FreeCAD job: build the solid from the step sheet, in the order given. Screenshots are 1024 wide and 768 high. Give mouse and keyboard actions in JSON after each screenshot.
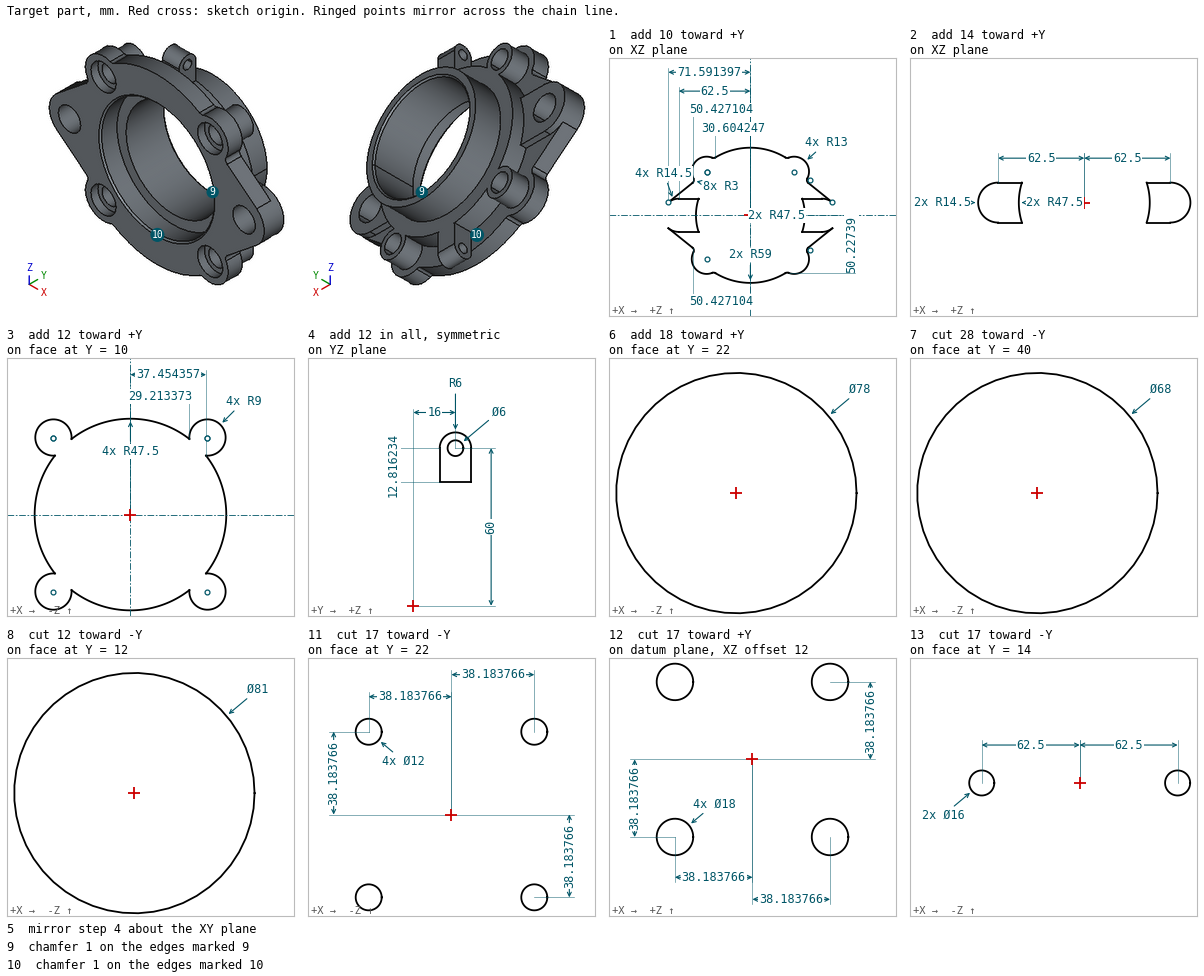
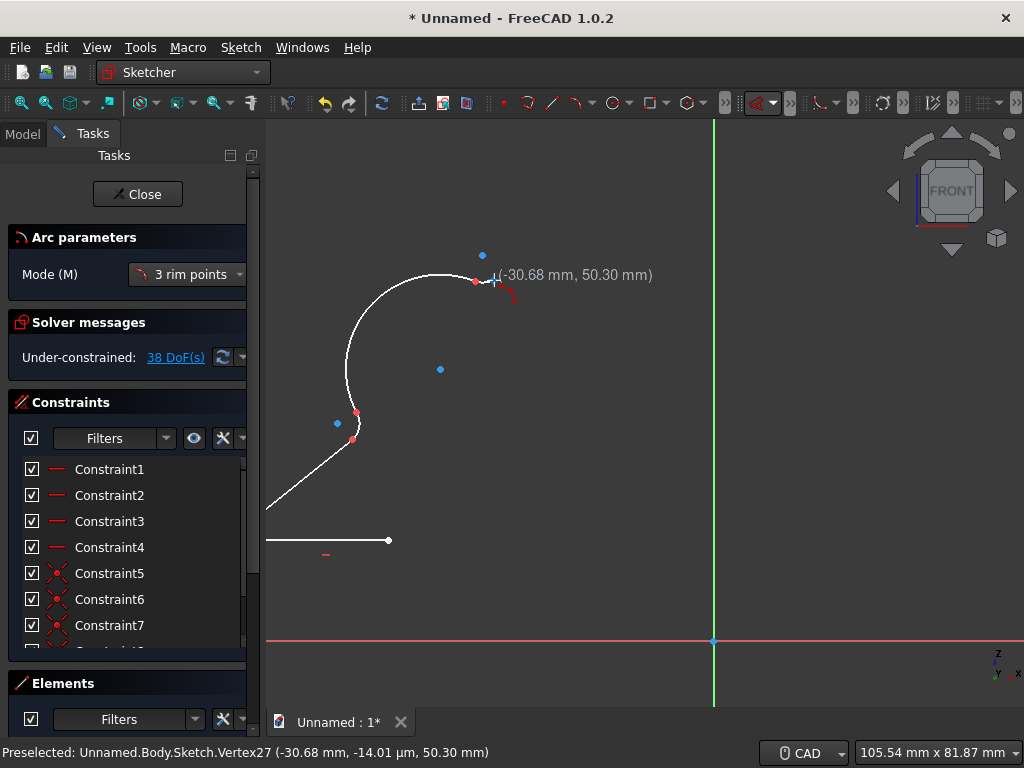
{"action": "scroll", "coordinate": [497, 280], "scroll_direction": "down", "scroll_amount": 5}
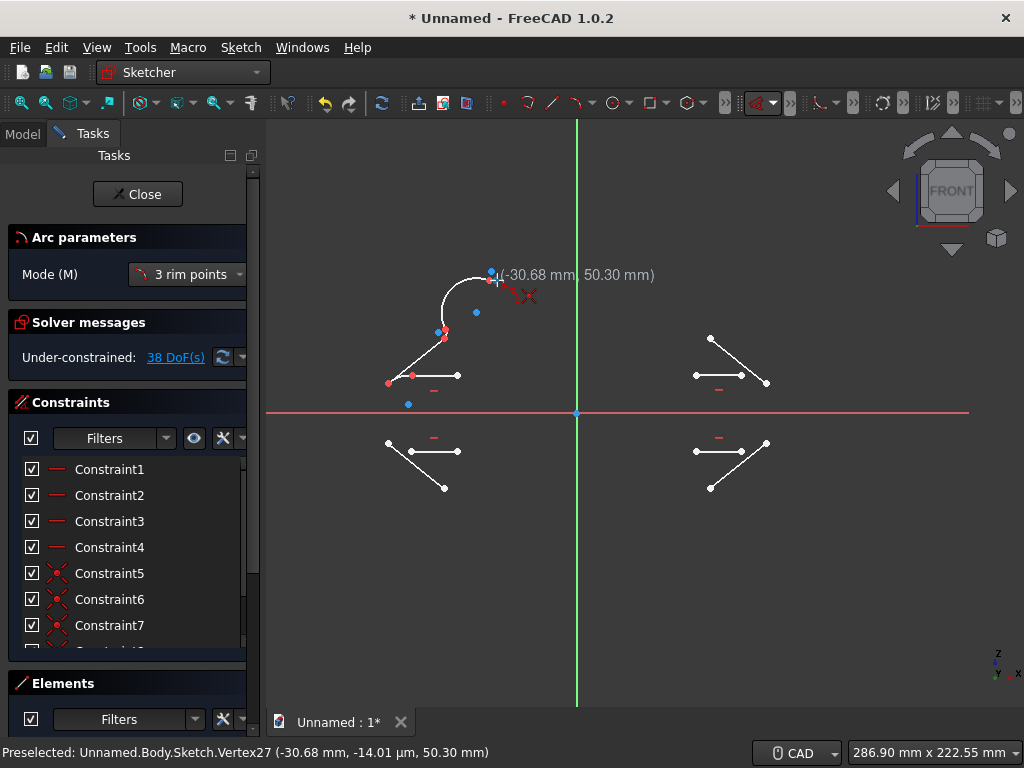
{"action": "left_click", "coordinate": [658, 280]}
{"action": "left_click", "coordinate": [594, 258]}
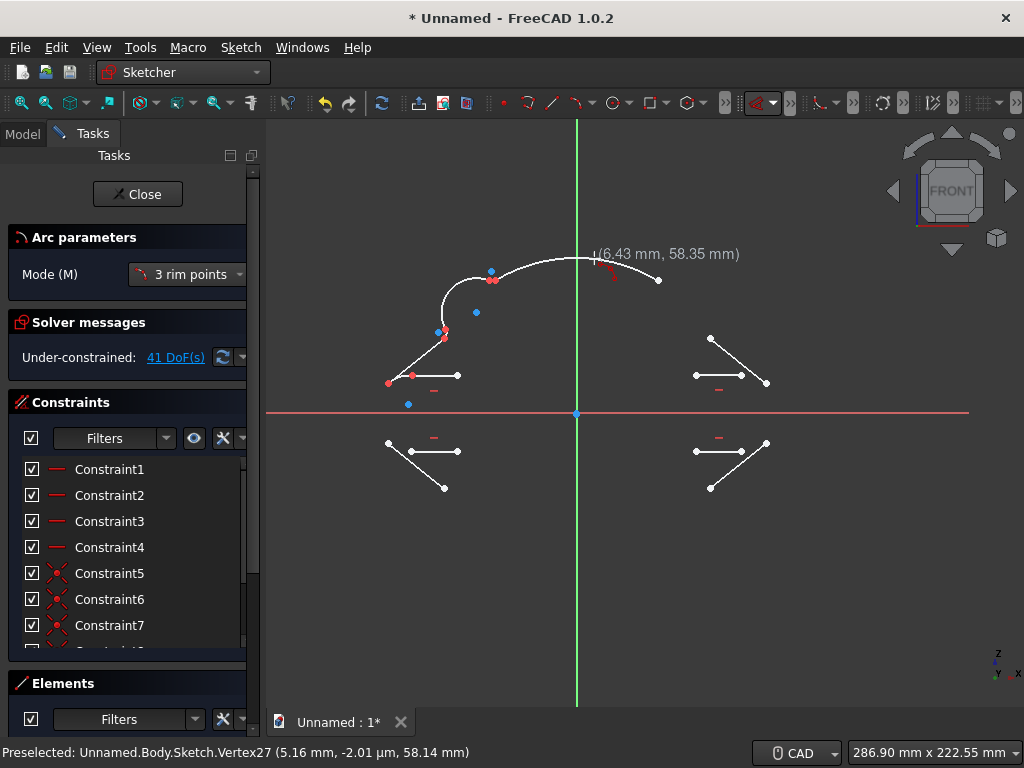
{"action": "left_click", "coordinate": [658, 281]}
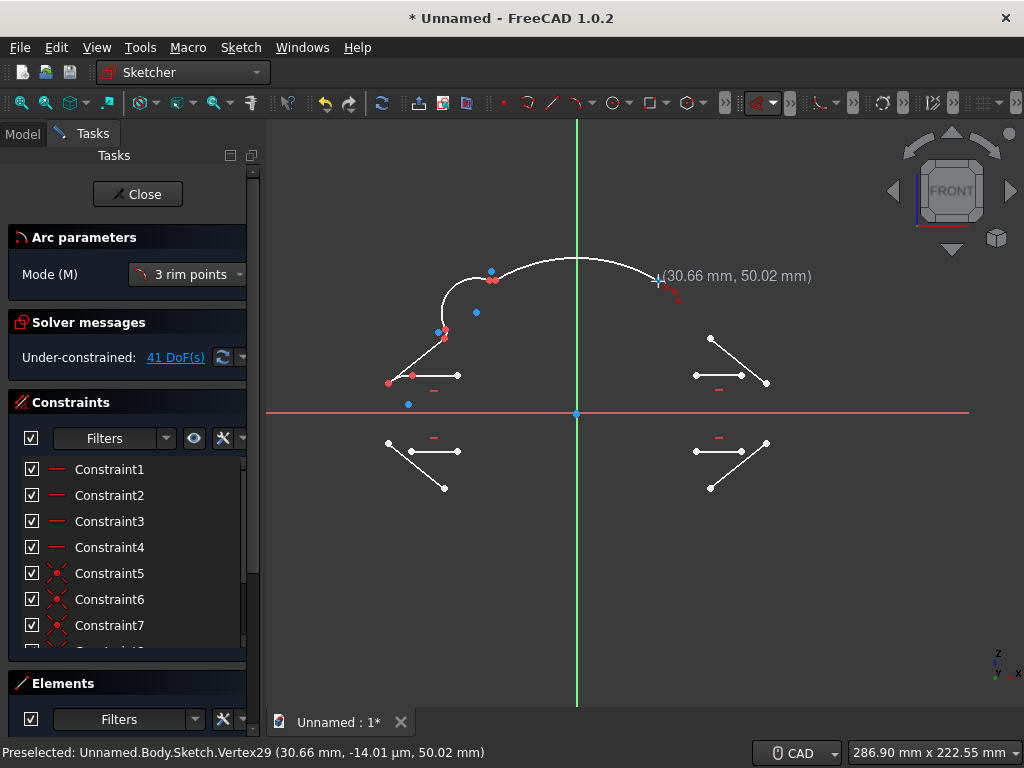
{"action": "scroll", "coordinate": [665, 280], "scroll_direction": "up", "scroll_amount": 5}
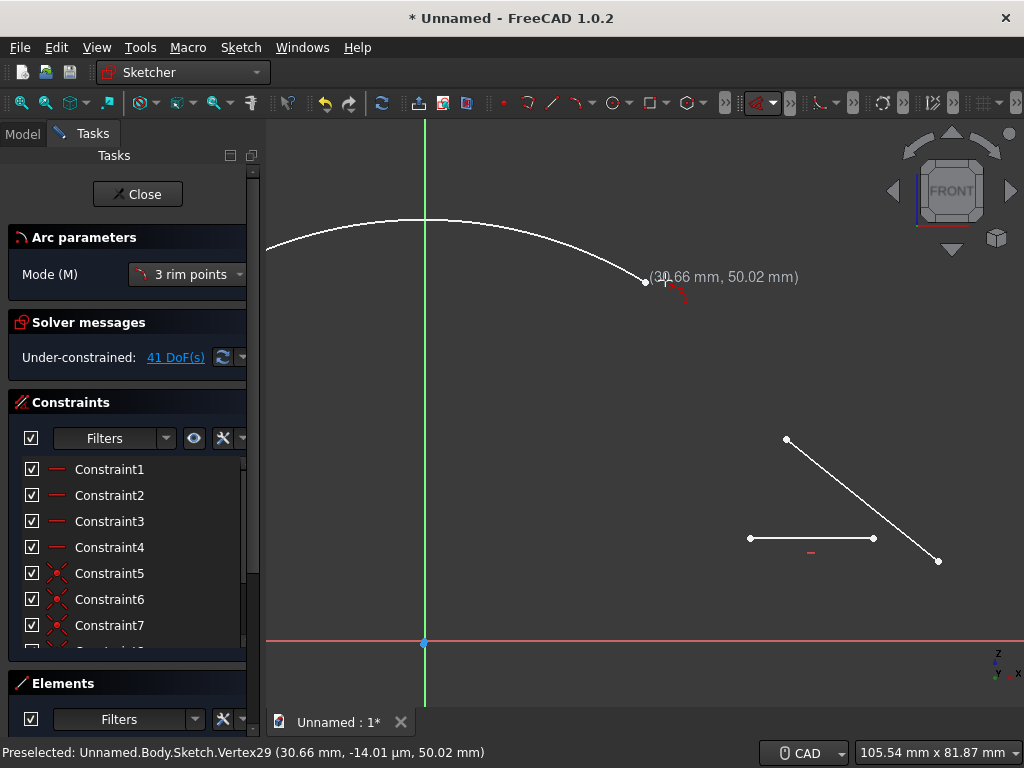
{"action": "left_click", "coordinate": [664, 281]}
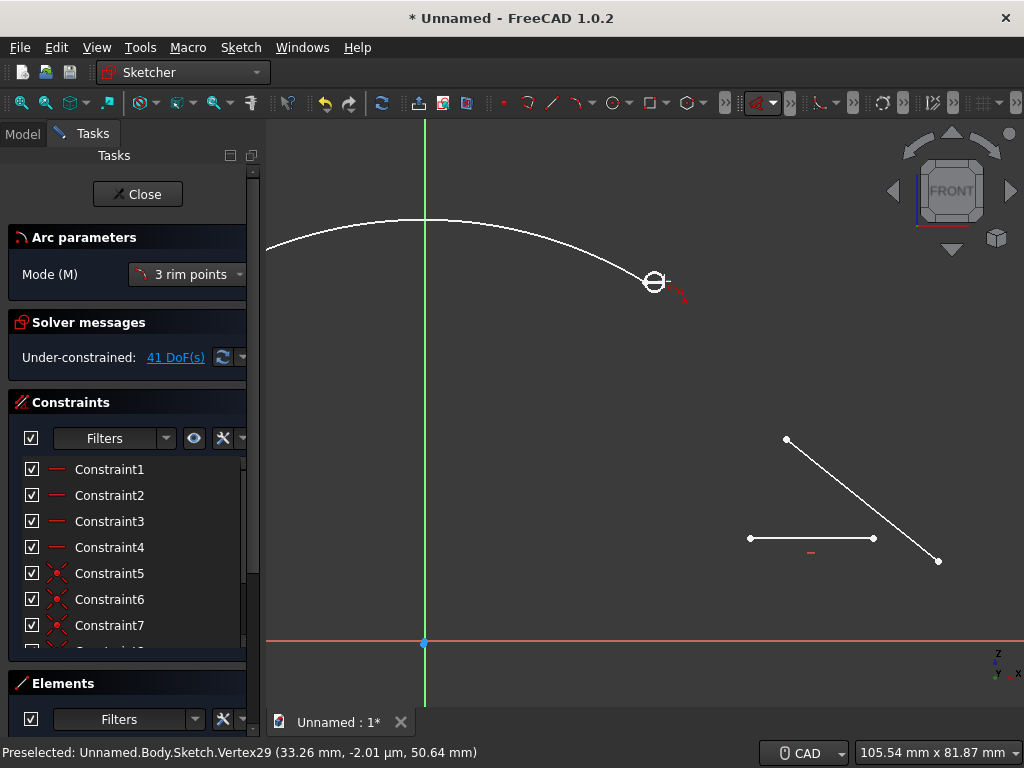
{"action": "scroll", "coordinate": [654, 282], "scroll_direction": "up", "scroll_amount": 10}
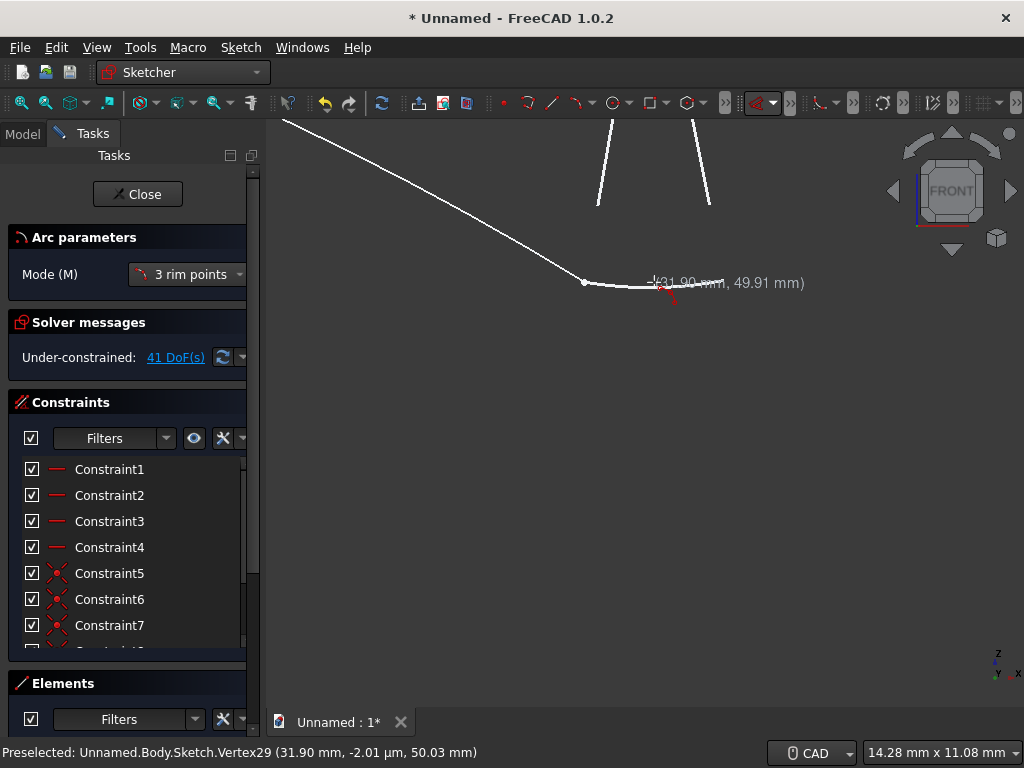
{"action": "left_click", "coordinate": [652, 282]}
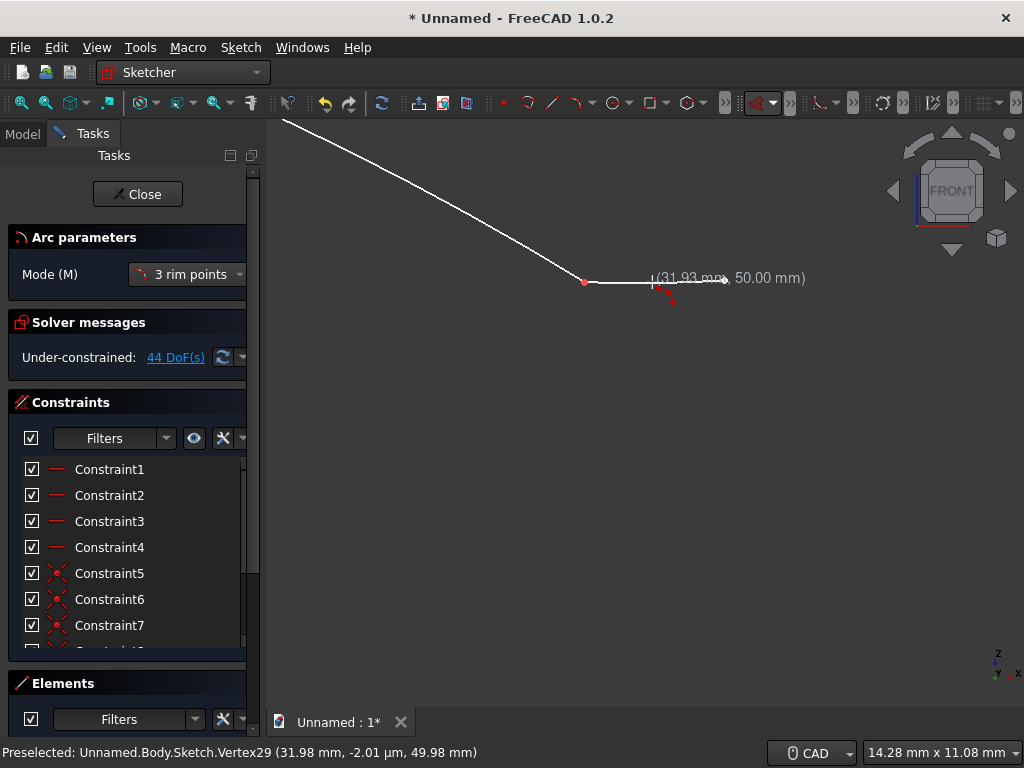
{"action": "scroll", "coordinate": [661, 281], "scroll_direction": "down", "scroll_amount": 15}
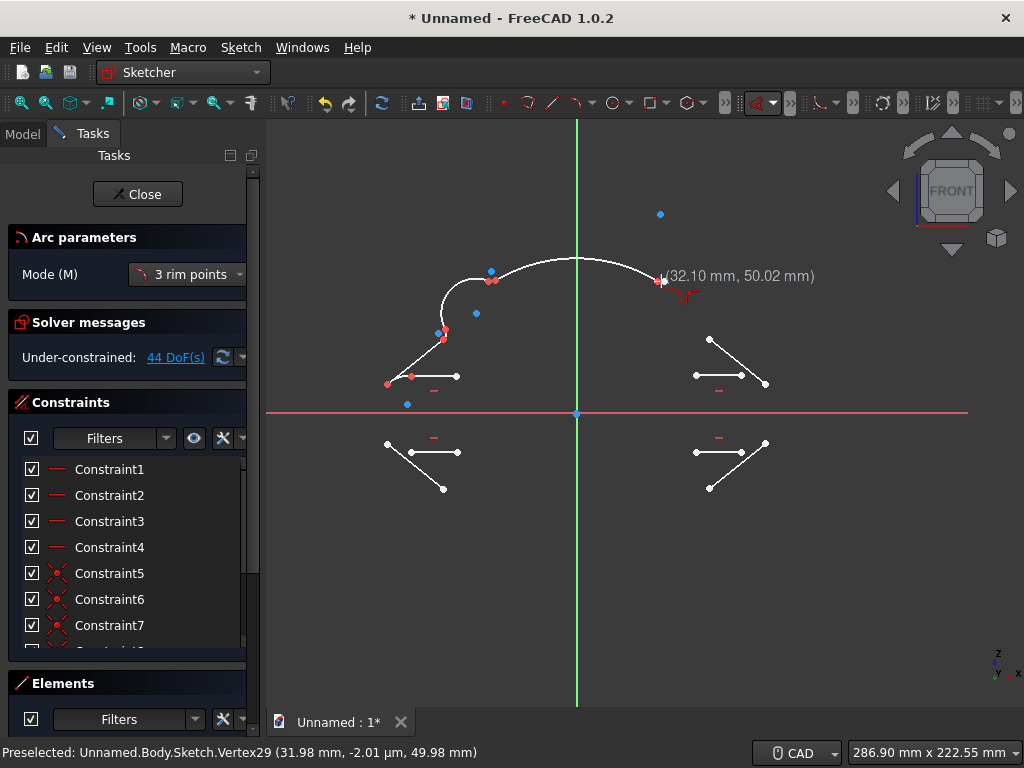
{"action": "scroll", "coordinate": [665, 281], "scroll_direction": "up", "scroll_amount": 5}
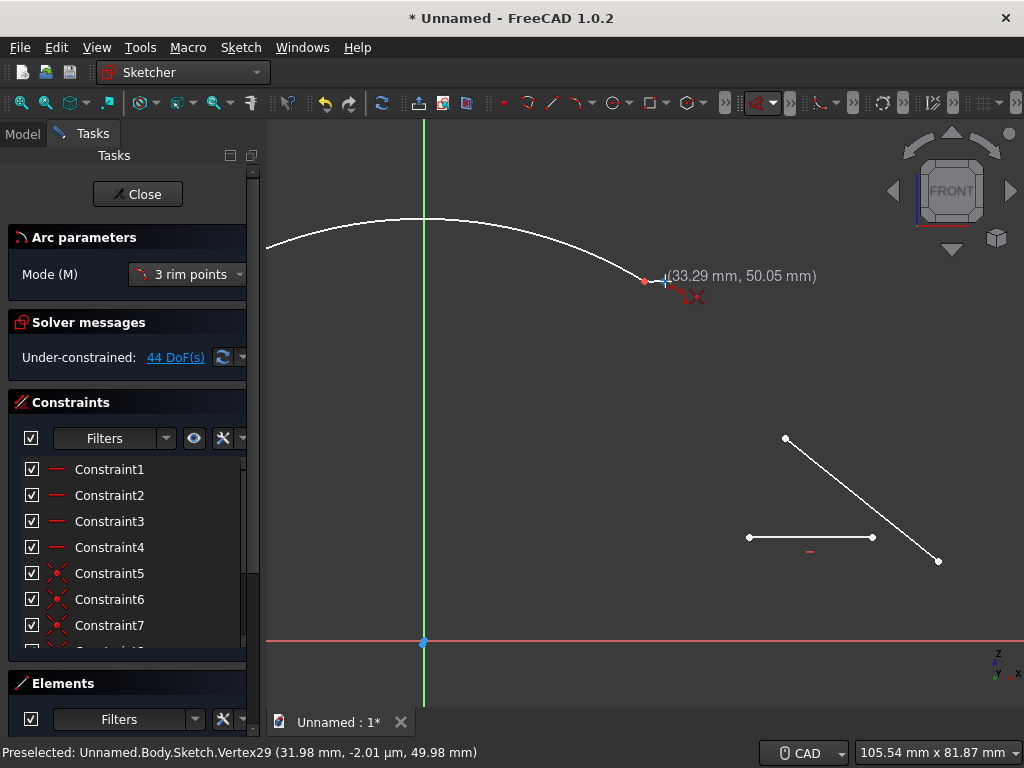
{"action": "left_click", "coordinate": [663, 281]}
{"action": "left_click", "coordinate": [781, 410]}
{"action": "left_click", "coordinate": [768, 304]}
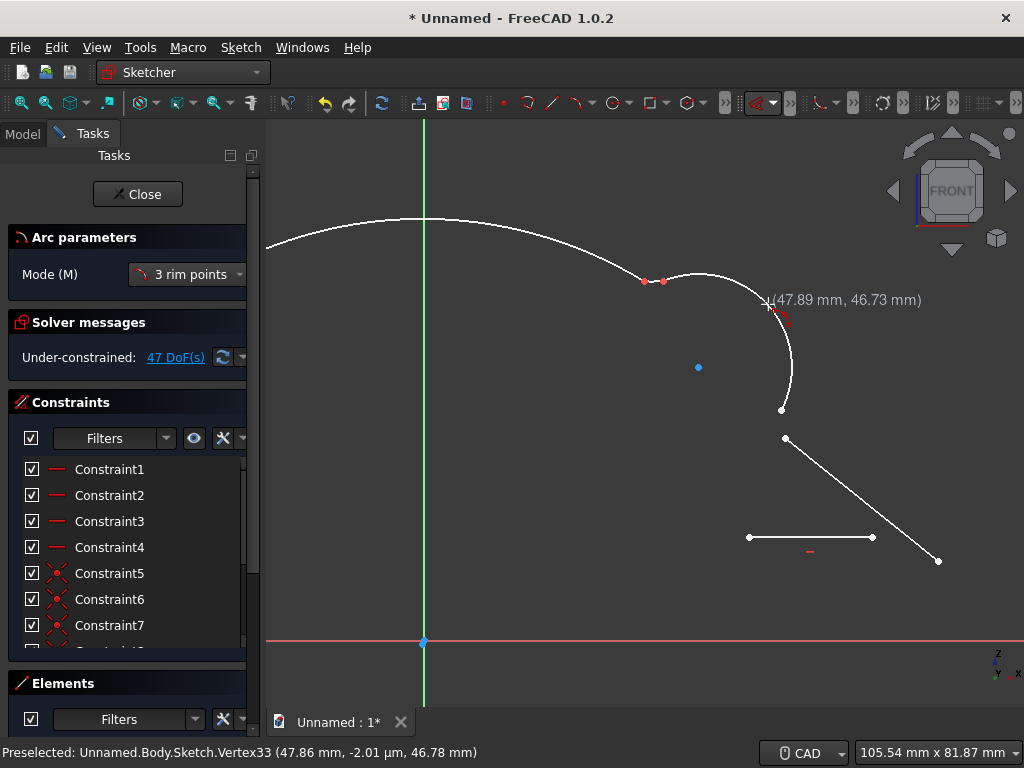
{"action": "left_click", "coordinate": [781, 411]}
{"action": "left_click", "coordinate": [786, 439]}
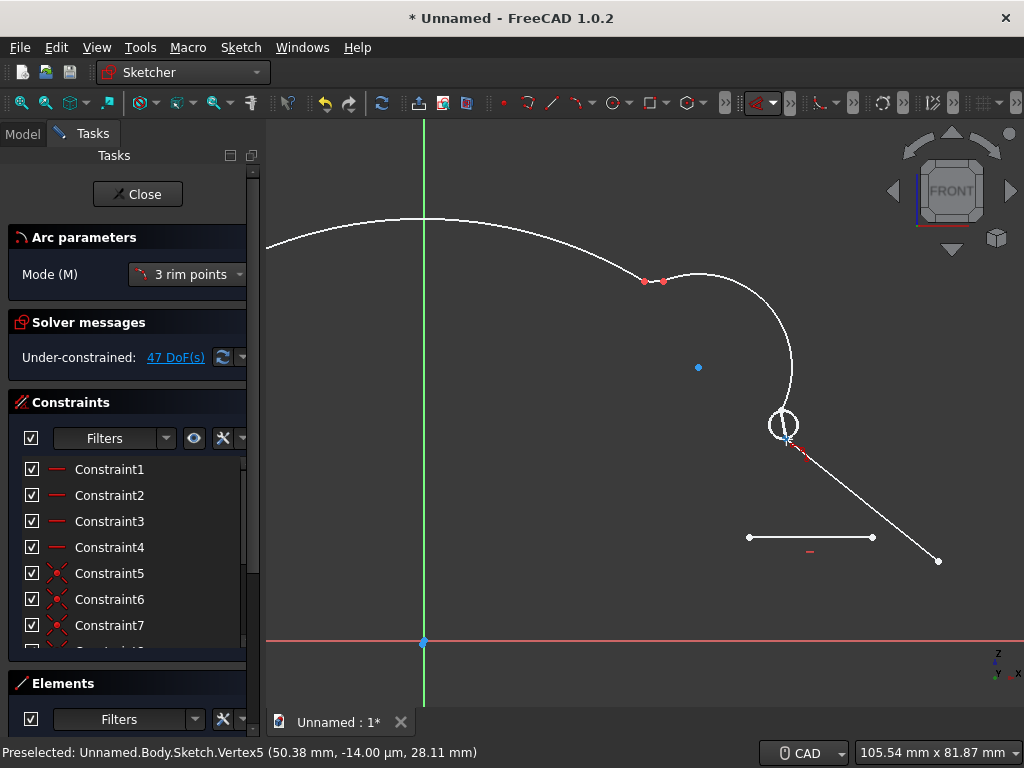
{"action": "scroll", "coordinate": [779, 425], "scroll_direction": "up", "scroll_amount": 6}